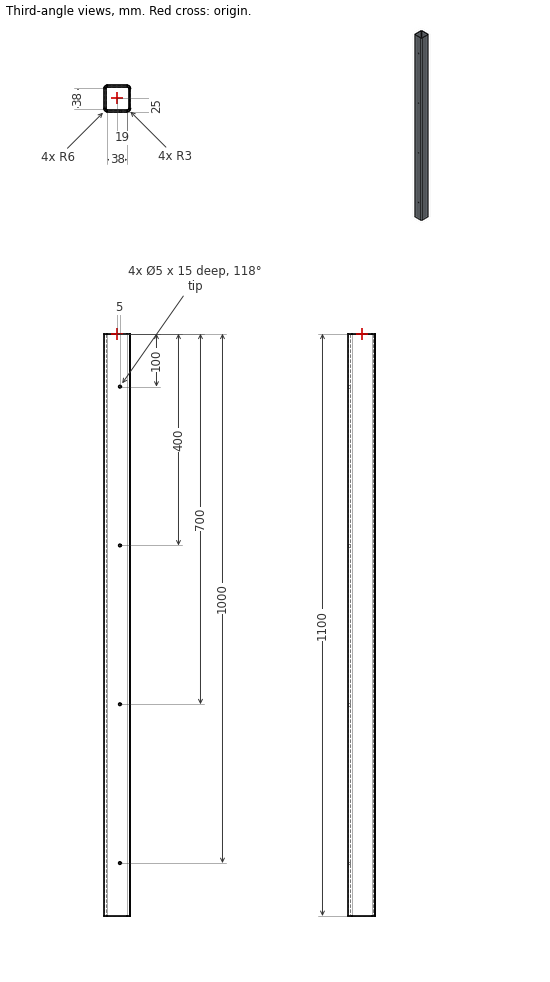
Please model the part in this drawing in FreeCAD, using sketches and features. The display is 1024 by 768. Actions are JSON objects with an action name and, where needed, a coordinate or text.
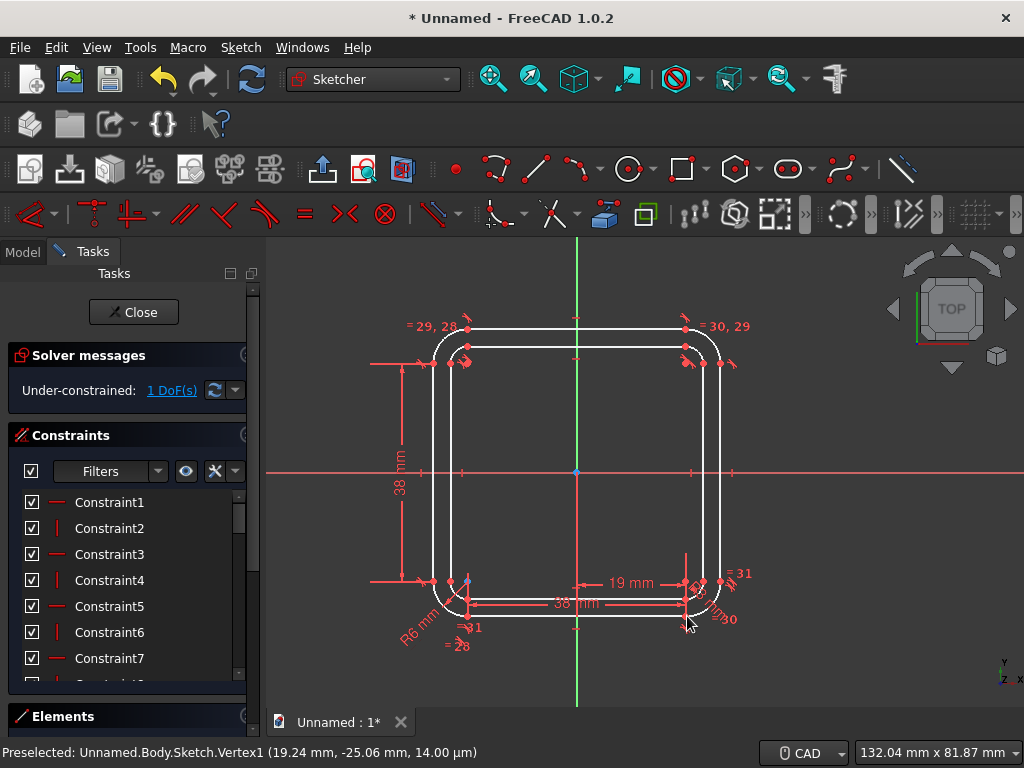
{"action": "left_click", "coordinate": [686, 616]}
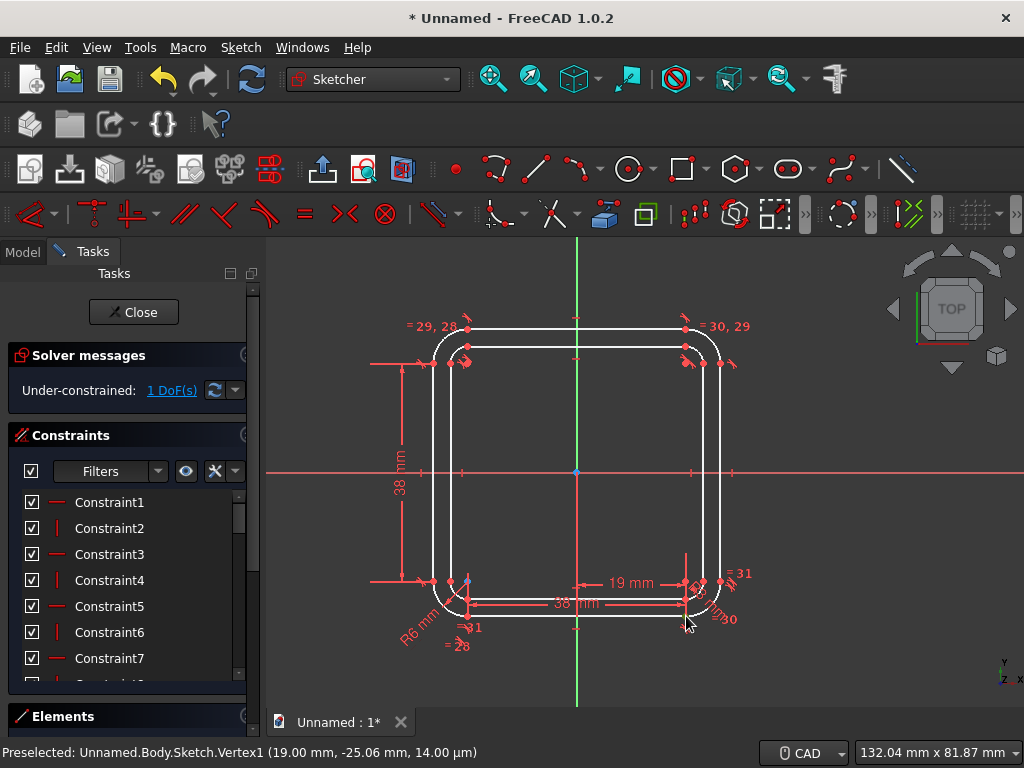
{"action": "key", "text": "i"}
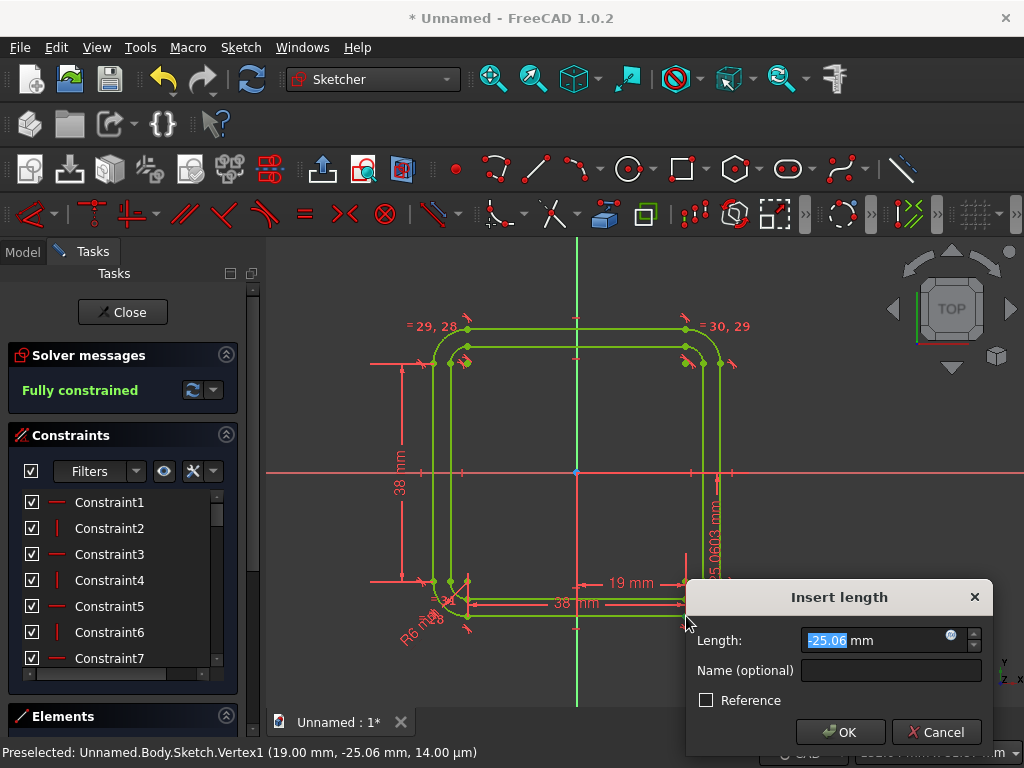
{"action": "type", "text": "-25"}
{"action": "key", "text": "Return"}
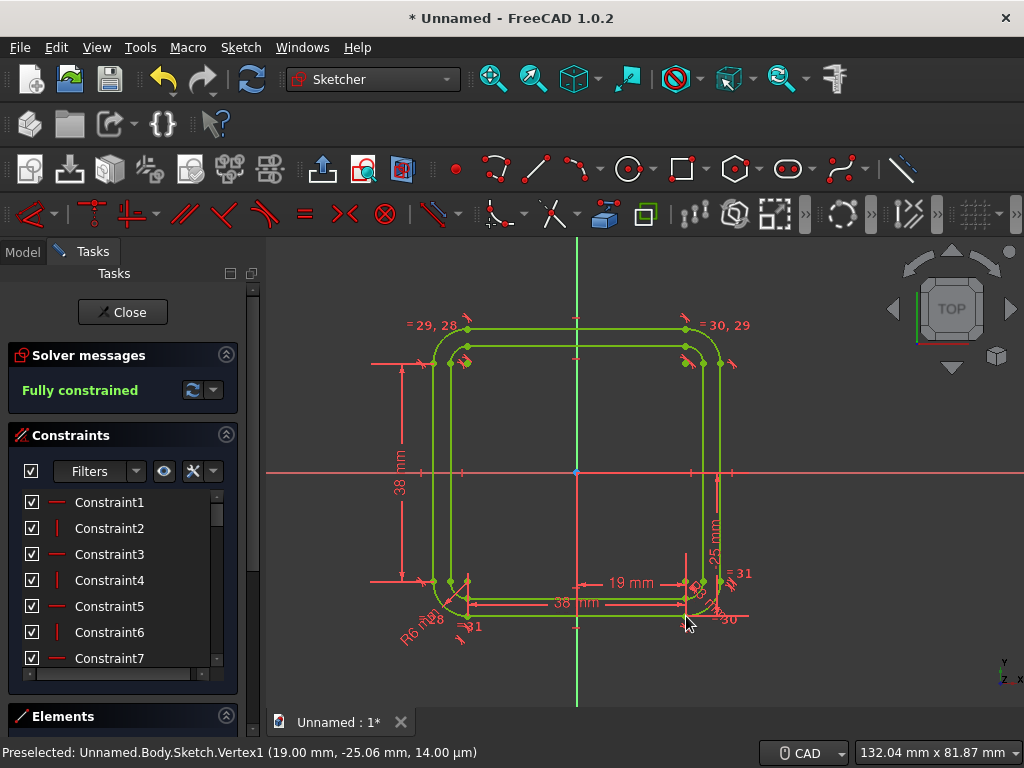
{"action": "left_click", "coordinate": [123, 312]}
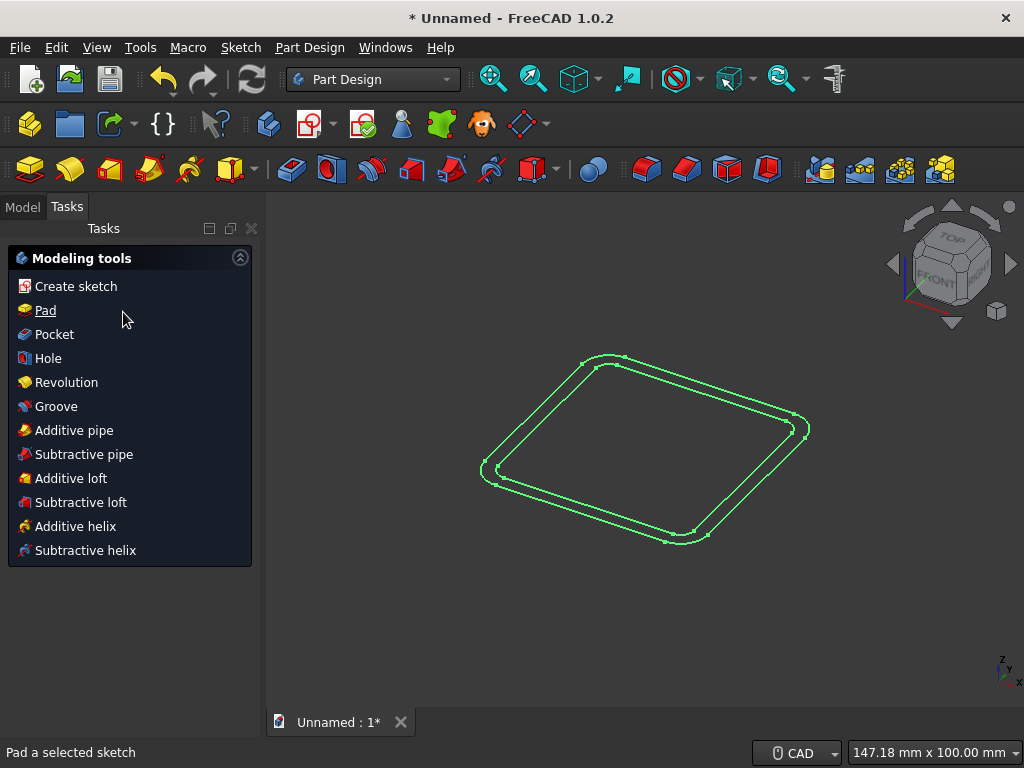
{"action": "left_click", "coordinate": [30, 170]}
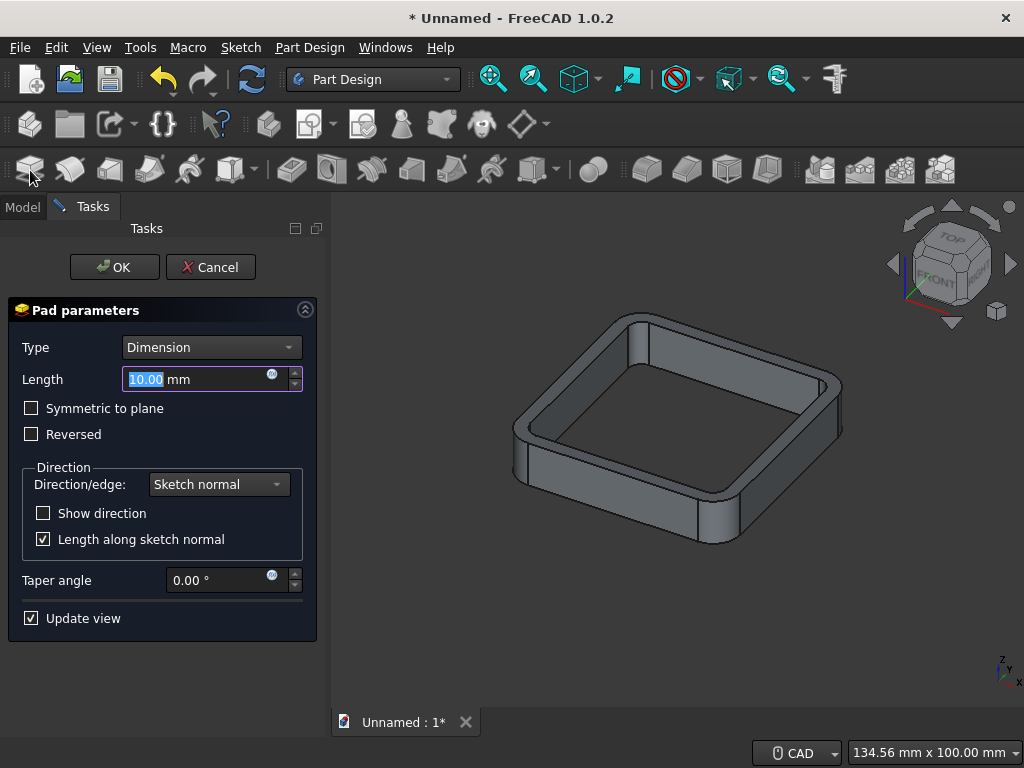
{"action": "type", "text": "1100"}
{"action": "key", "text": "Tab"}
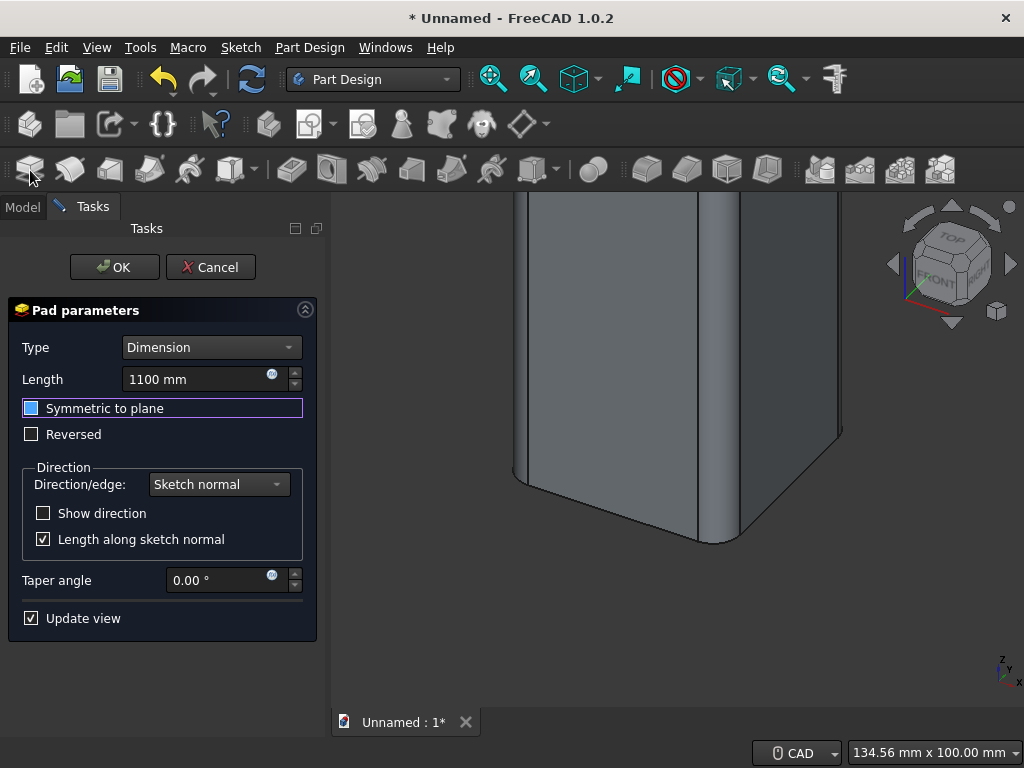
{"action": "left_click", "coordinate": [30, 434]}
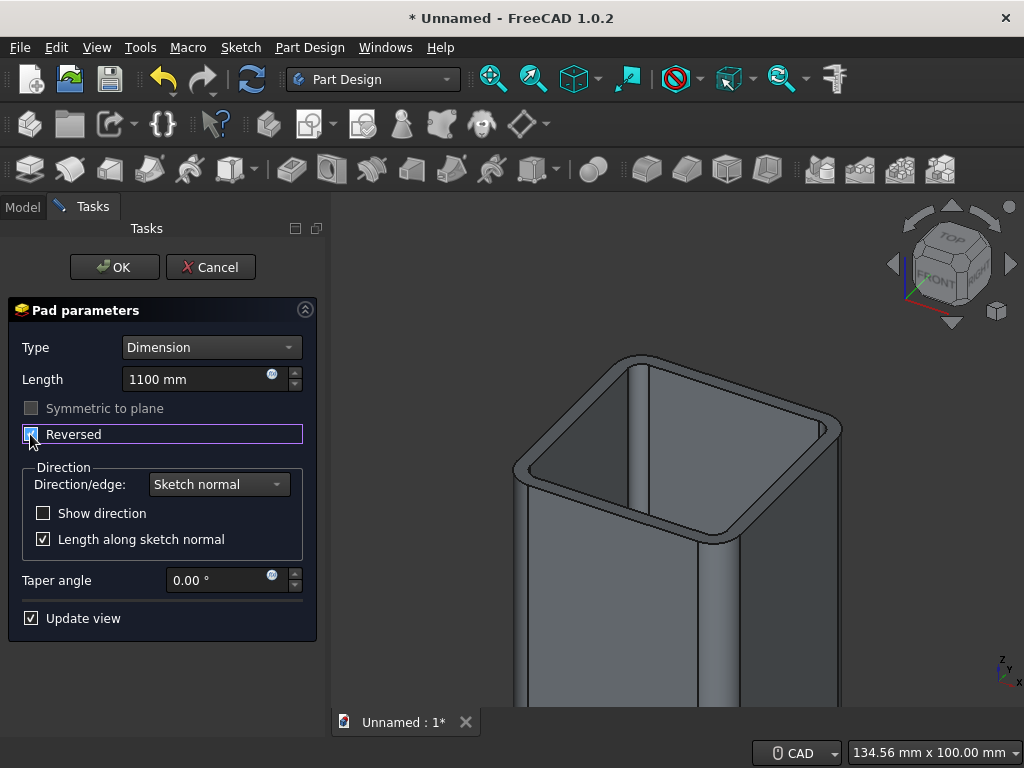
{"action": "left_click", "coordinate": [115, 267]}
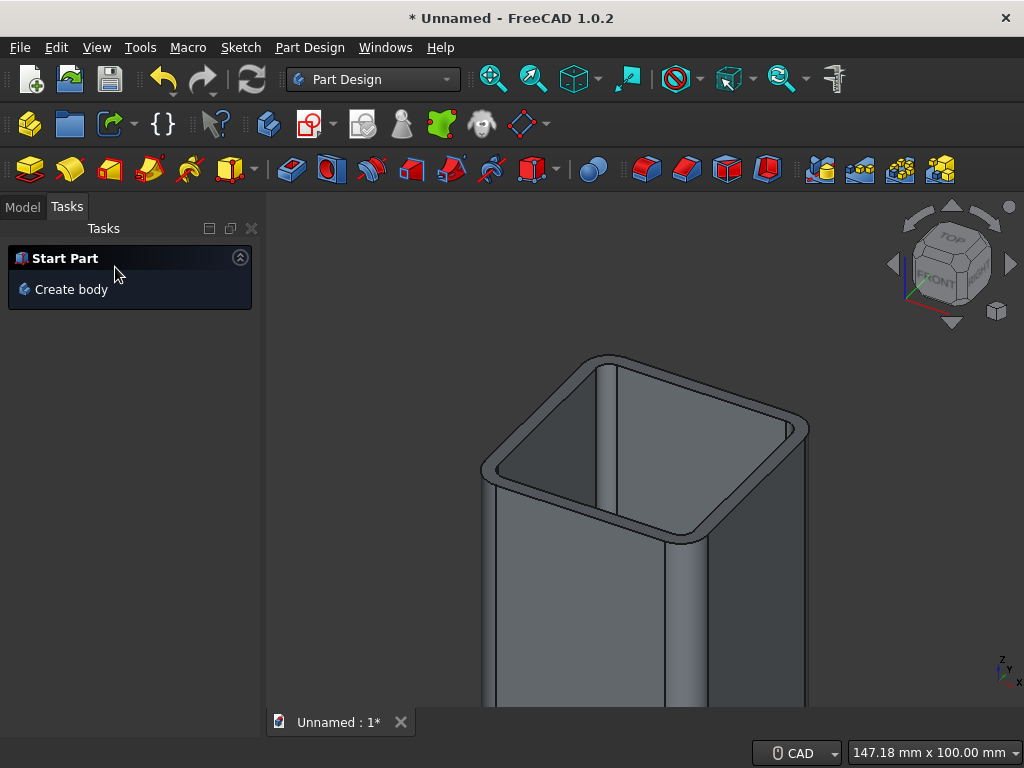
{"action": "key", "text": "v f"}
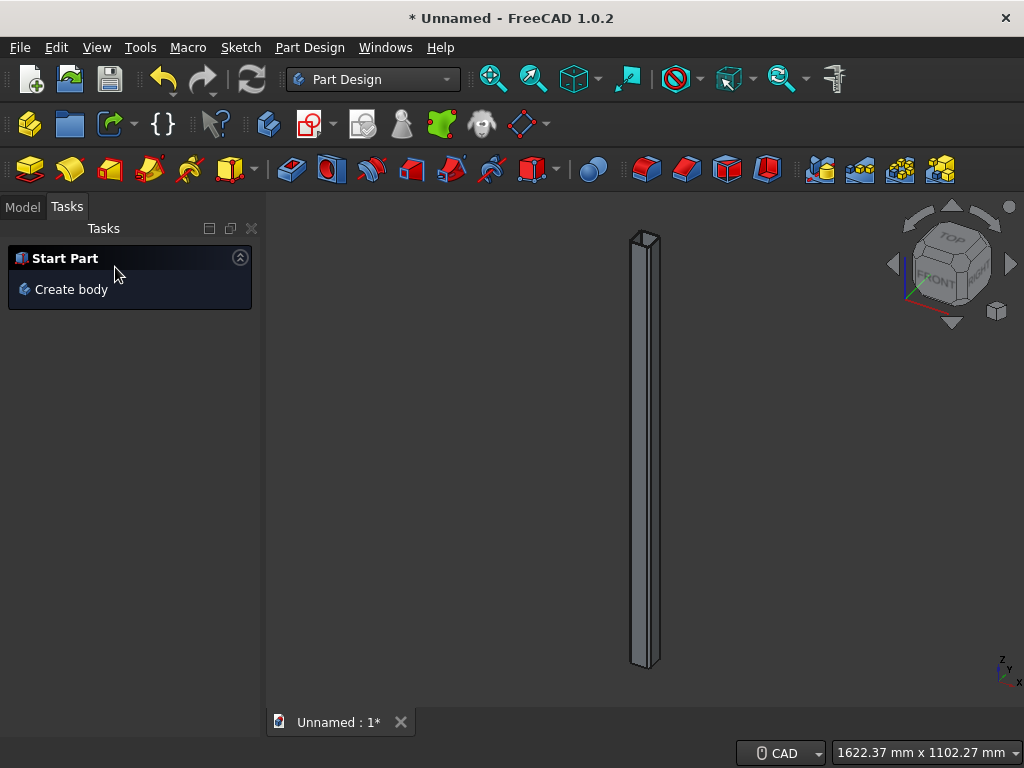
{"action": "left_click", "coordinate": [637, 273]}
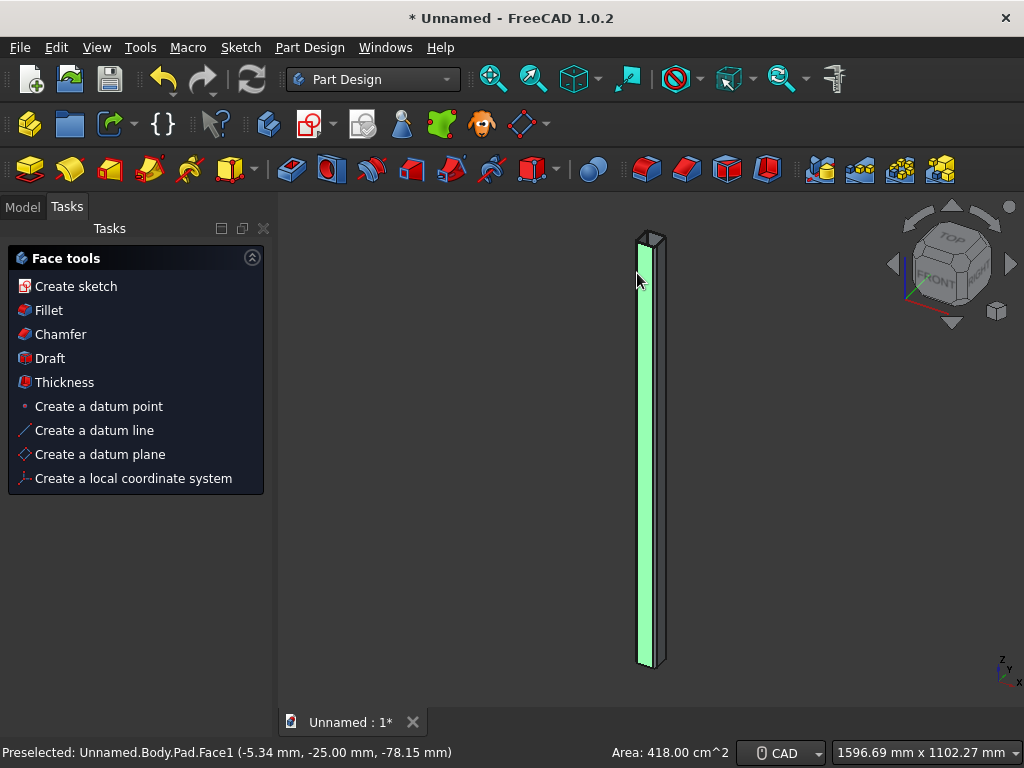
{"action": "left_click", "coordinate": [310, 124]}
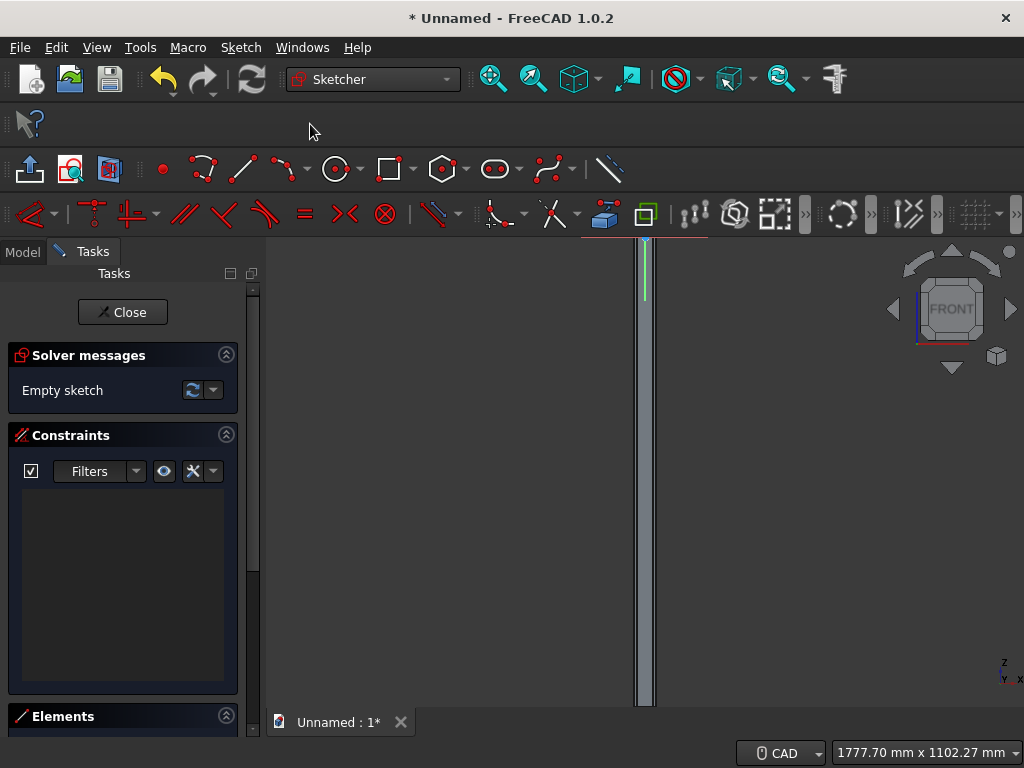
{"action": "scroll", "coordinate": [434, 514], "scroll_direction": "down", "scroll_amount": 2}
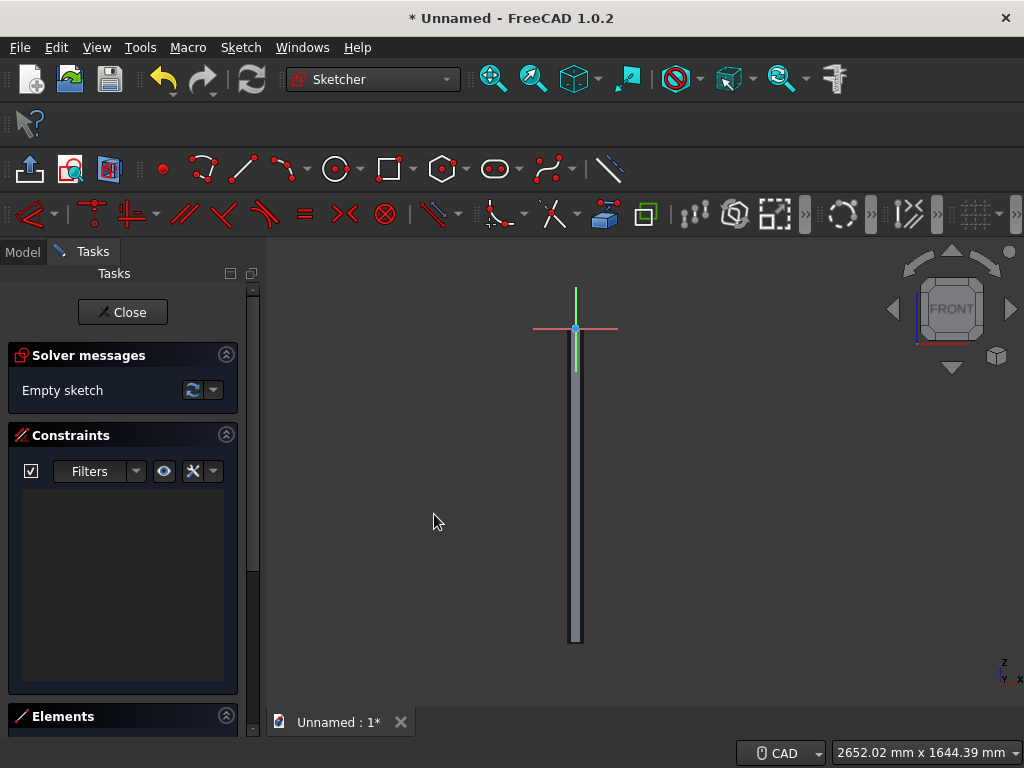
{"action": "key", "text": "g c"}